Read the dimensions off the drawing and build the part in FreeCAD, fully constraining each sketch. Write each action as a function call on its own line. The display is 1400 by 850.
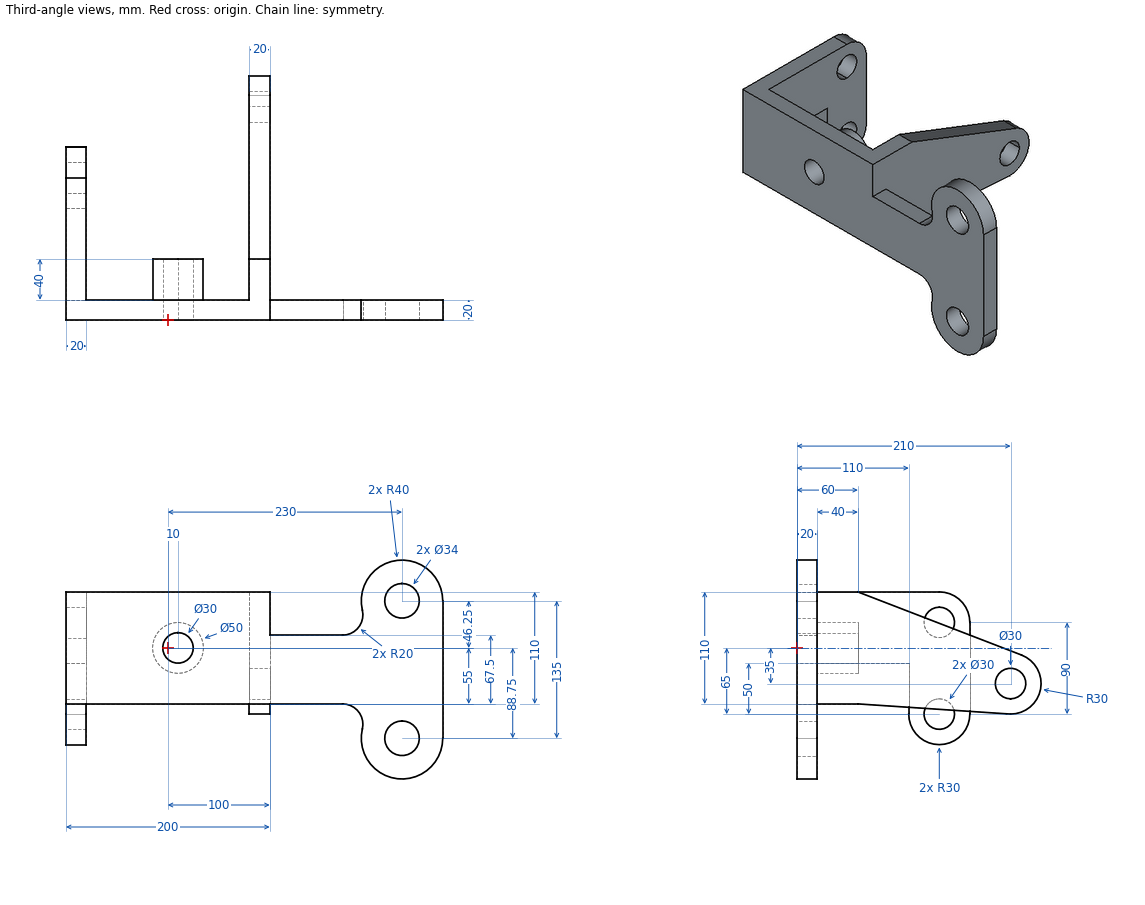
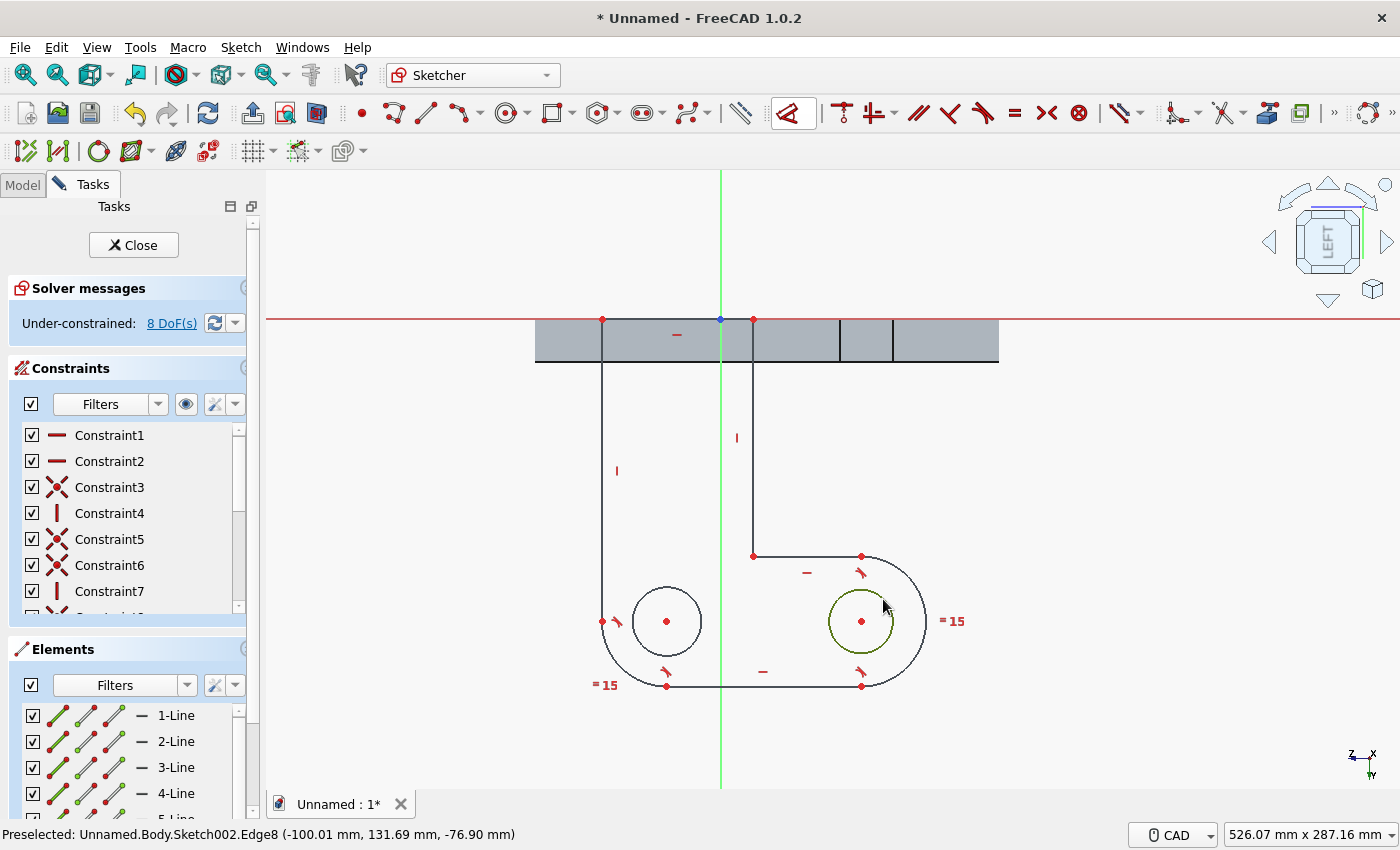
click(691, 597)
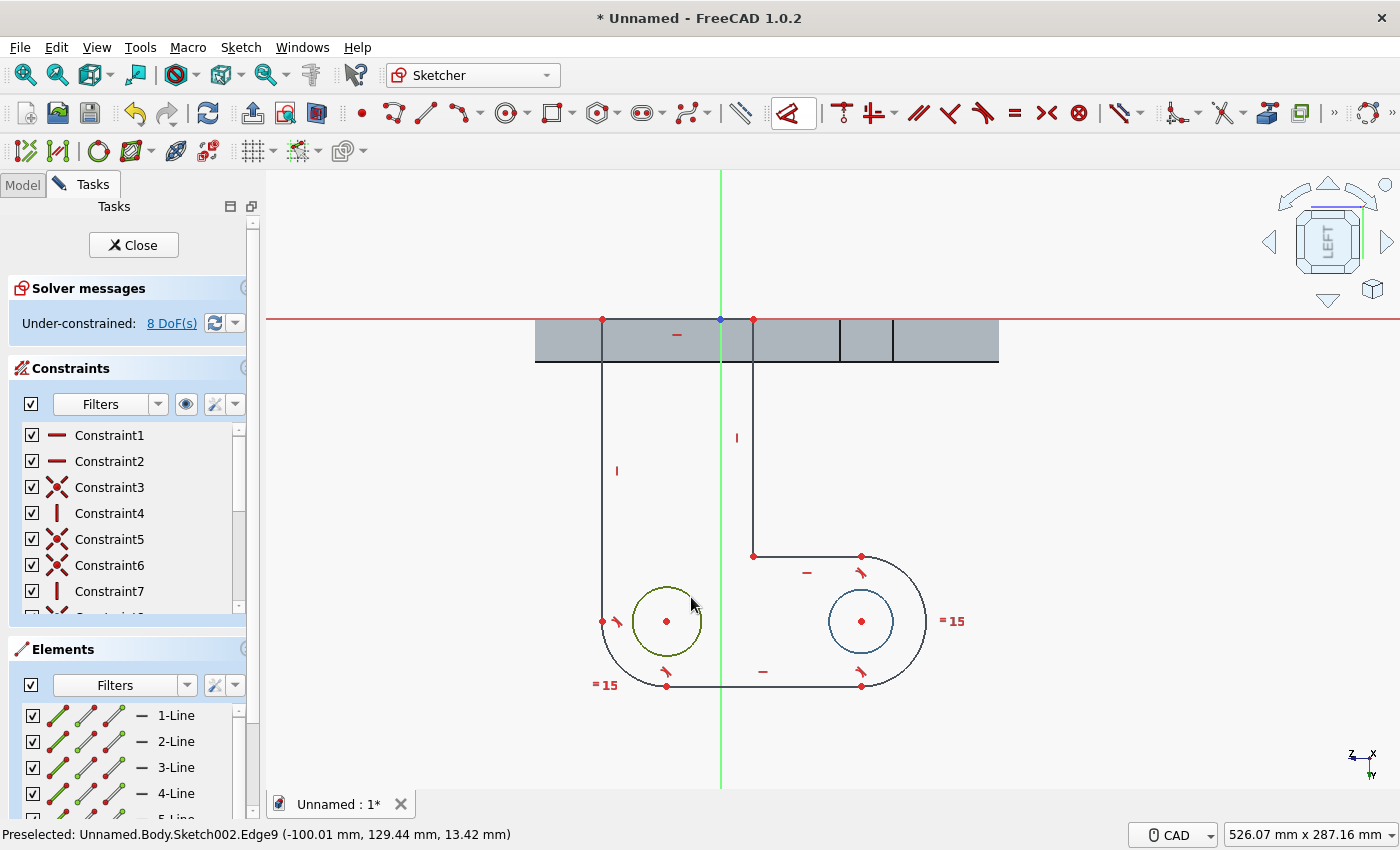
key(e)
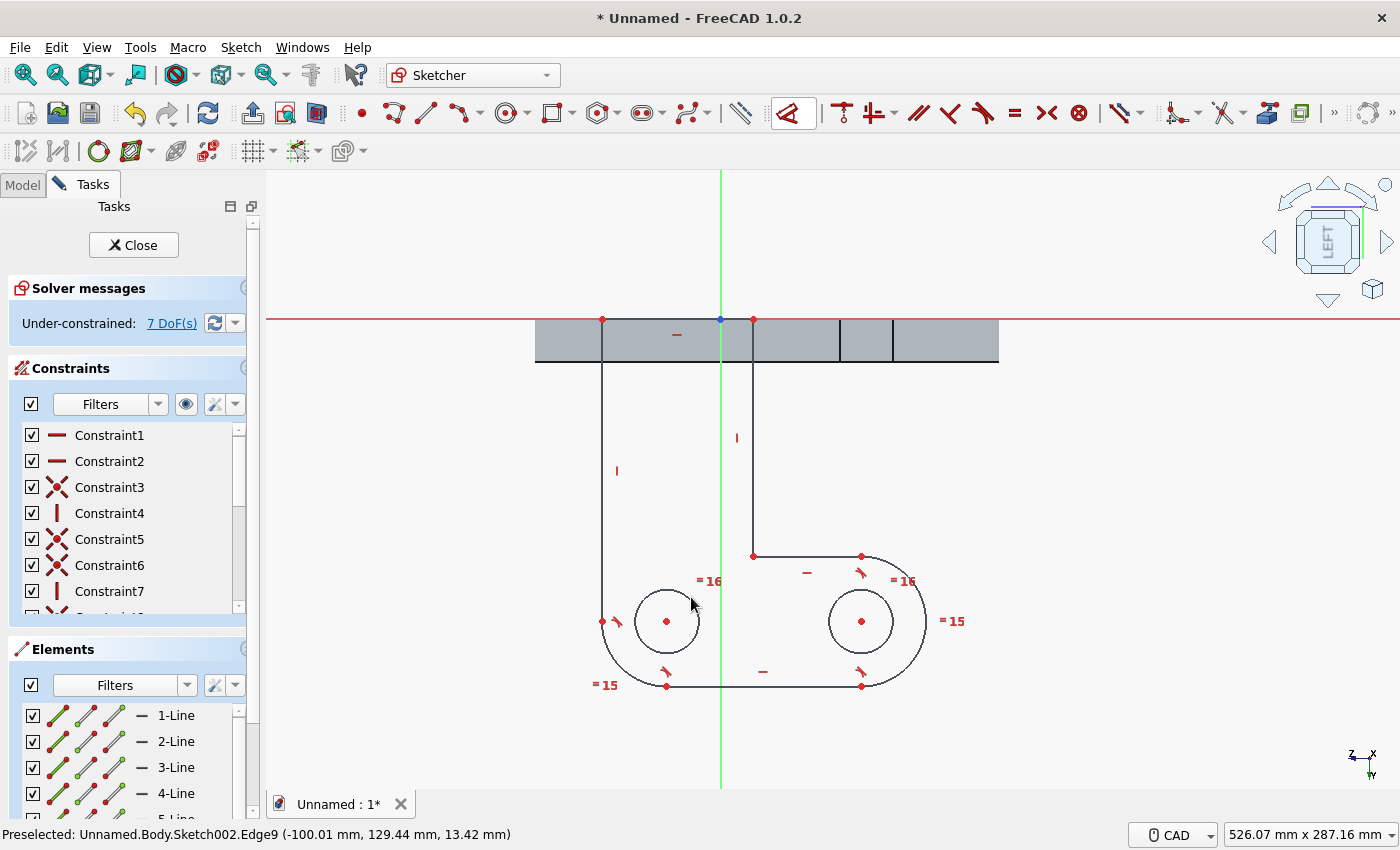
click(914, 660)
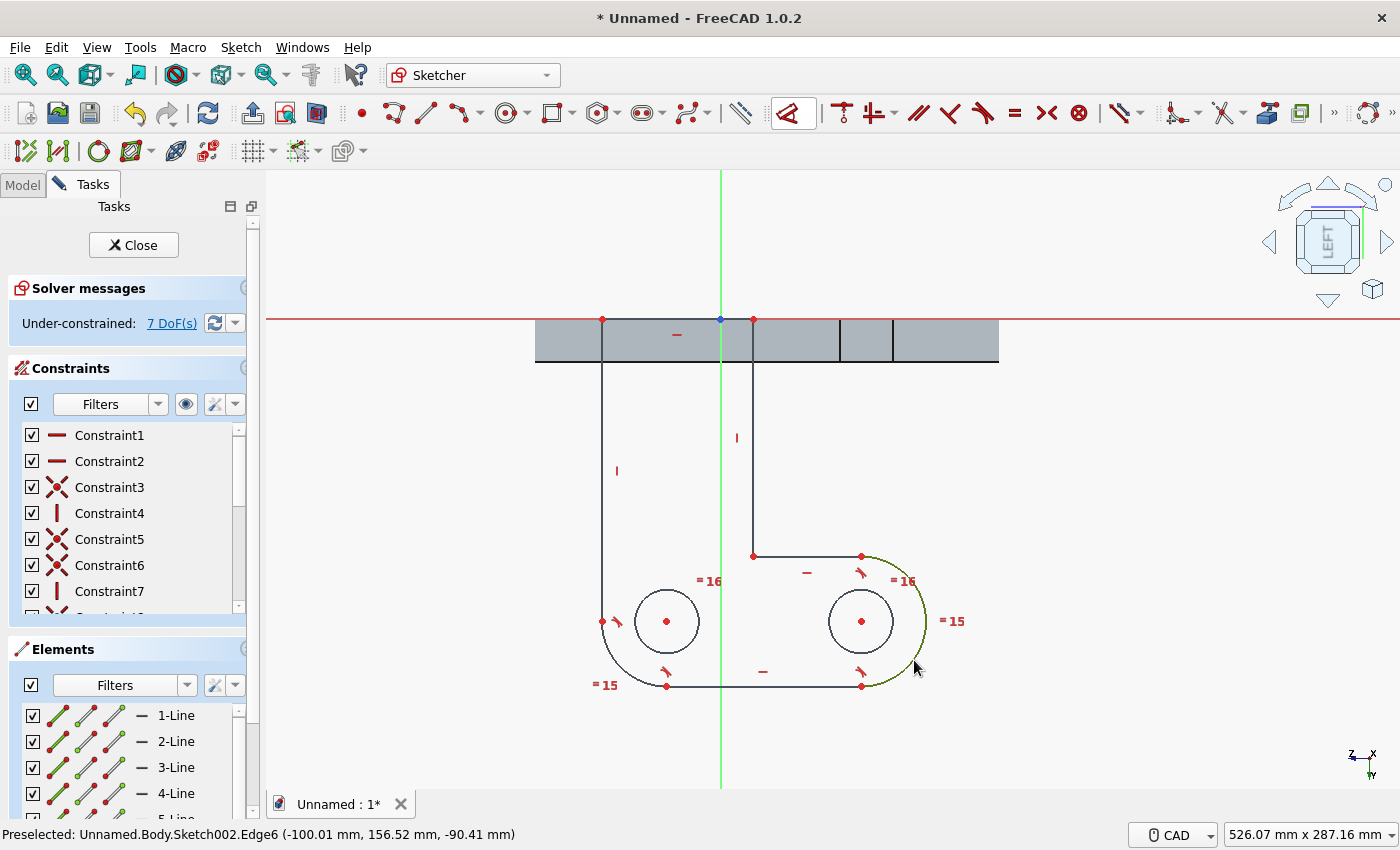
click(810, 114)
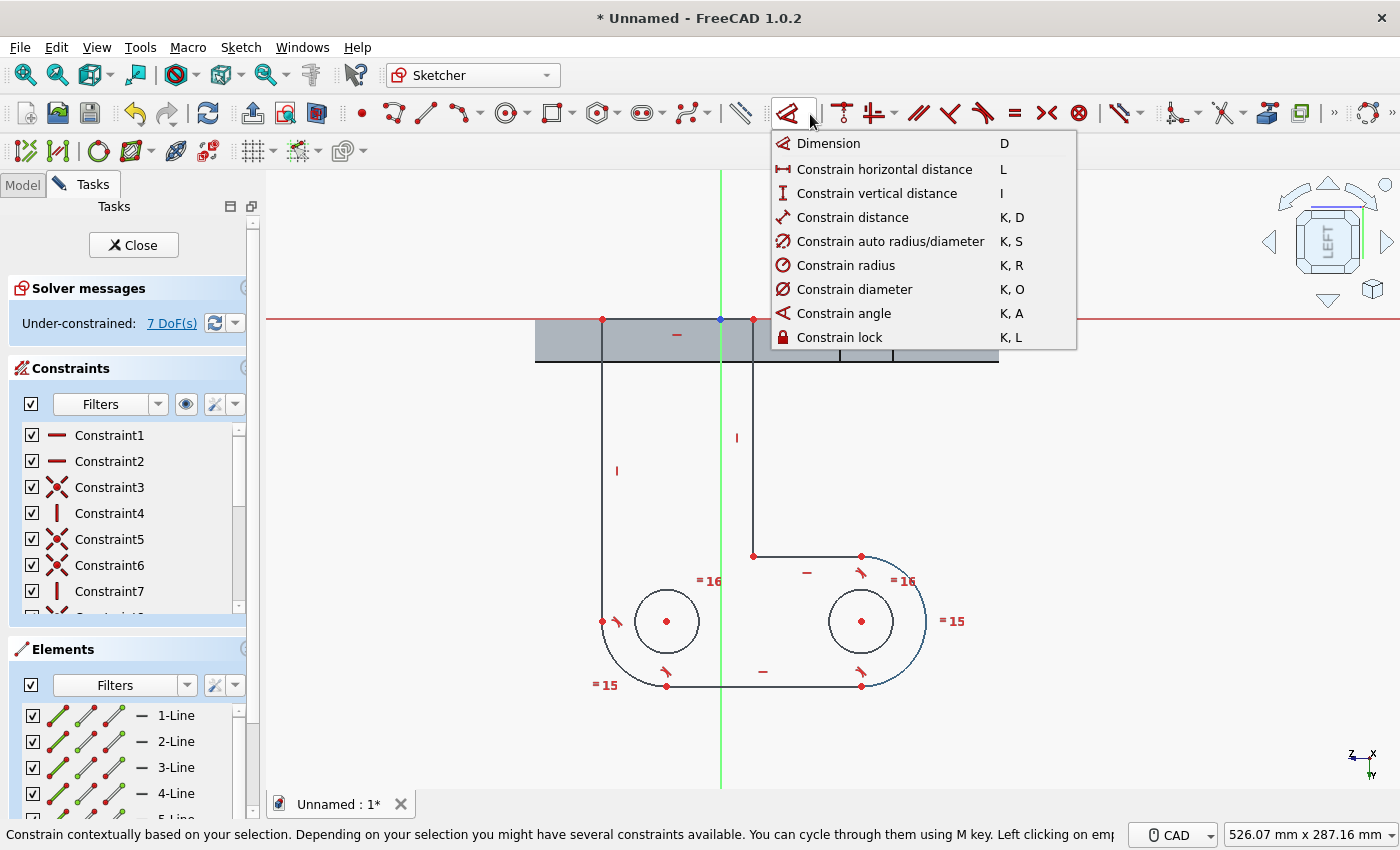
click(924, 265)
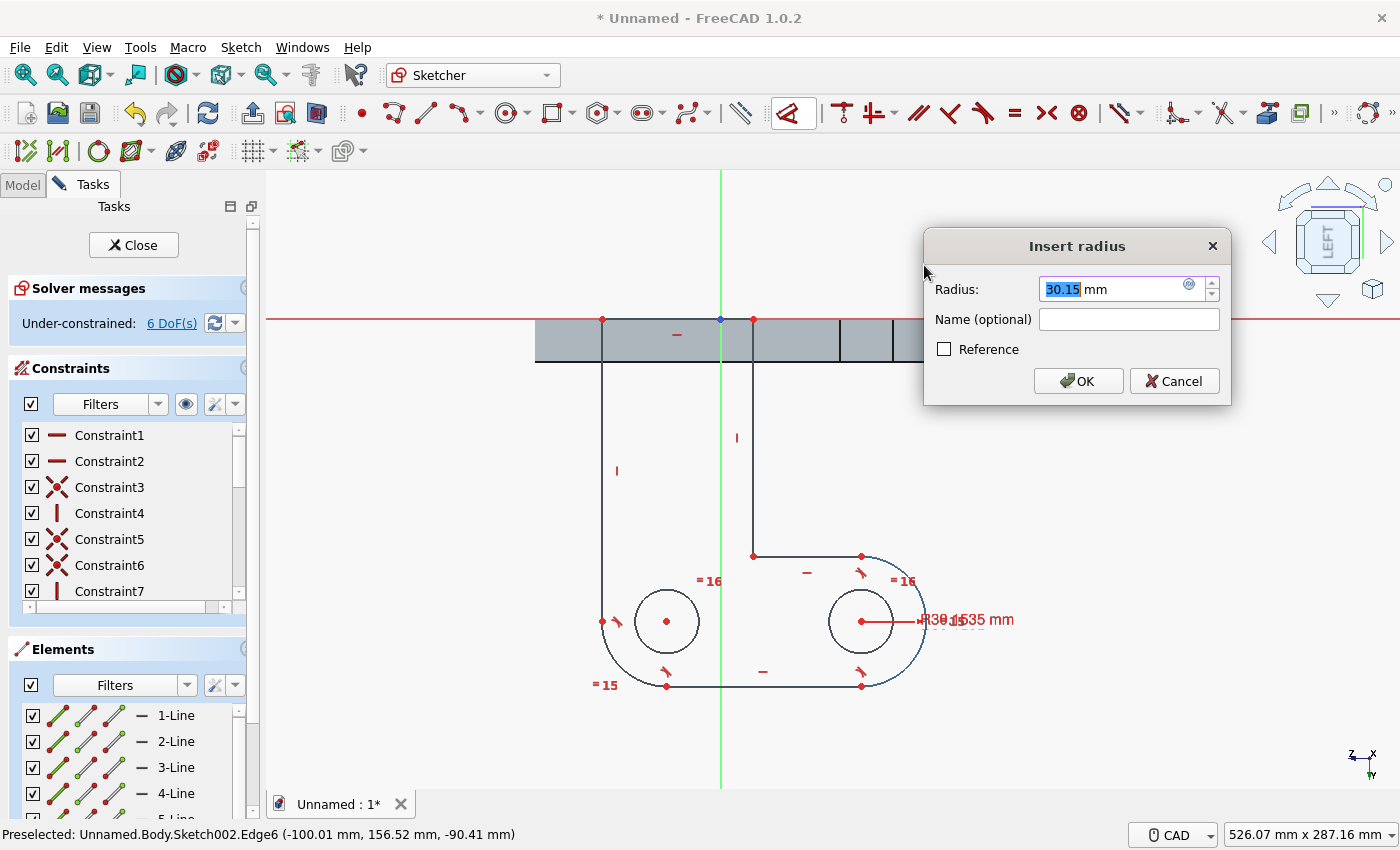
text(30)
key(Return)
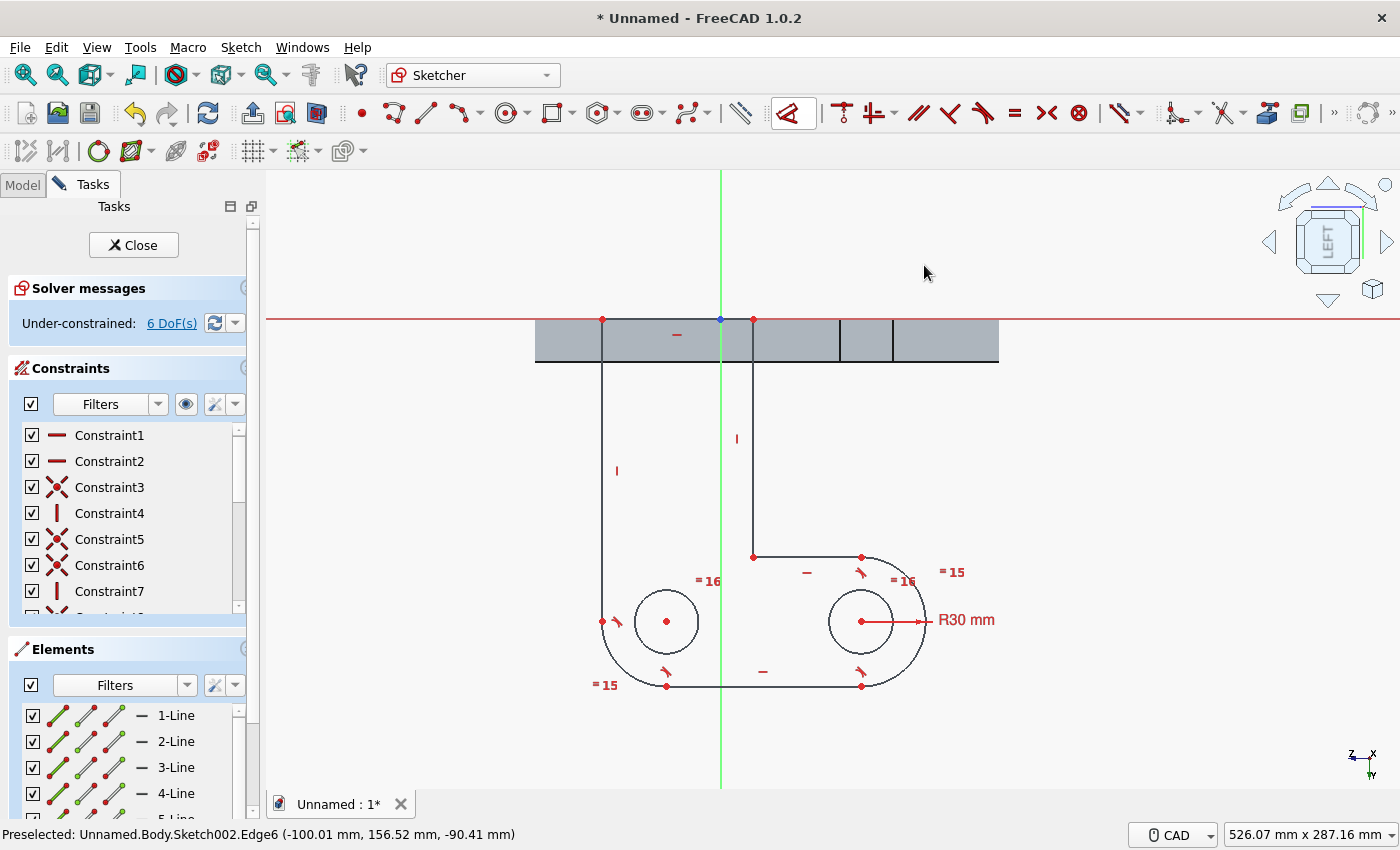
click(883, 599)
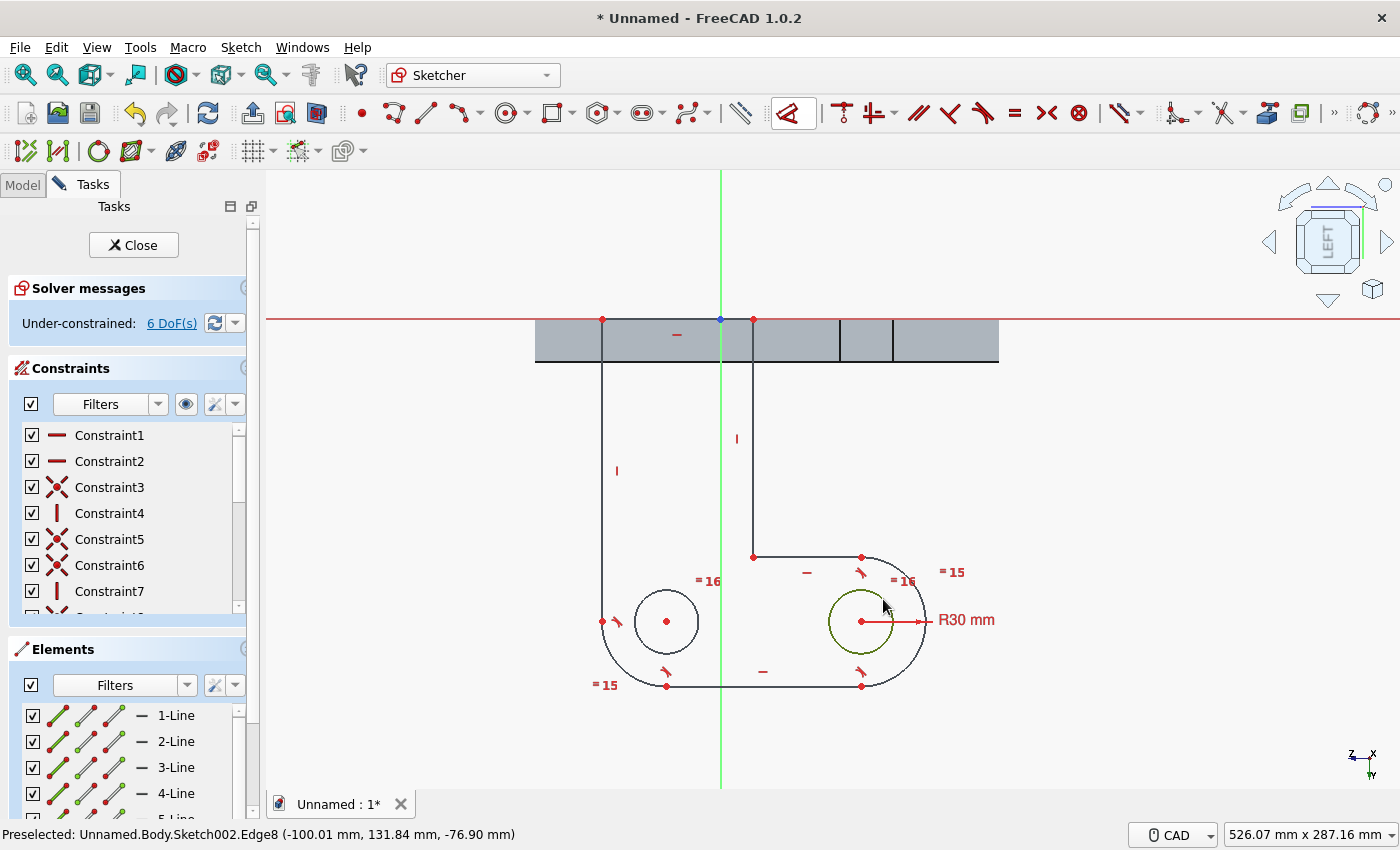
key(k)
key(o)